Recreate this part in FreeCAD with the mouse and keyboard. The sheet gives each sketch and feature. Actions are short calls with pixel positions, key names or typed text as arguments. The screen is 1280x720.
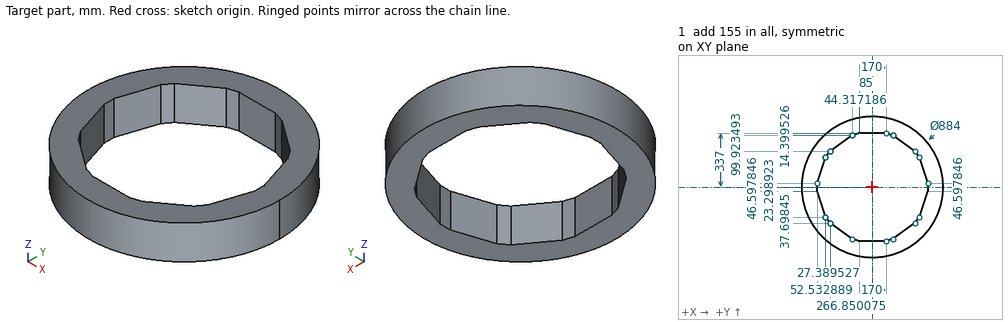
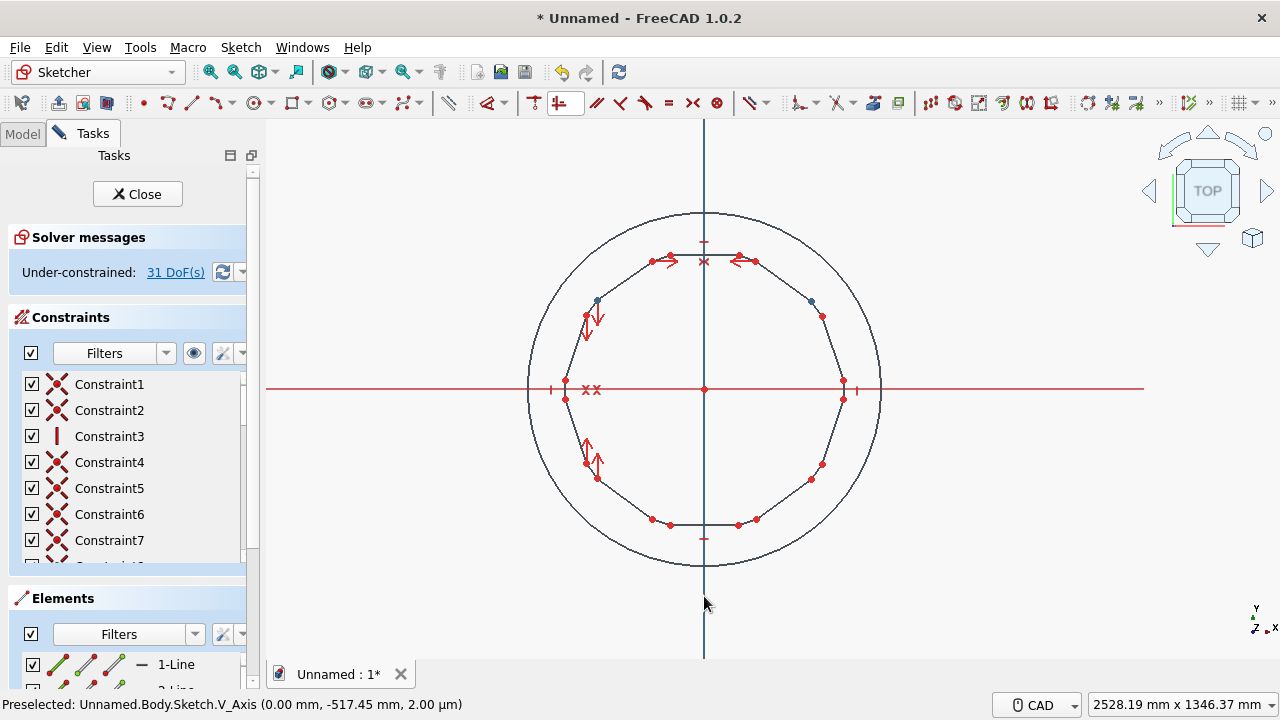
key(s)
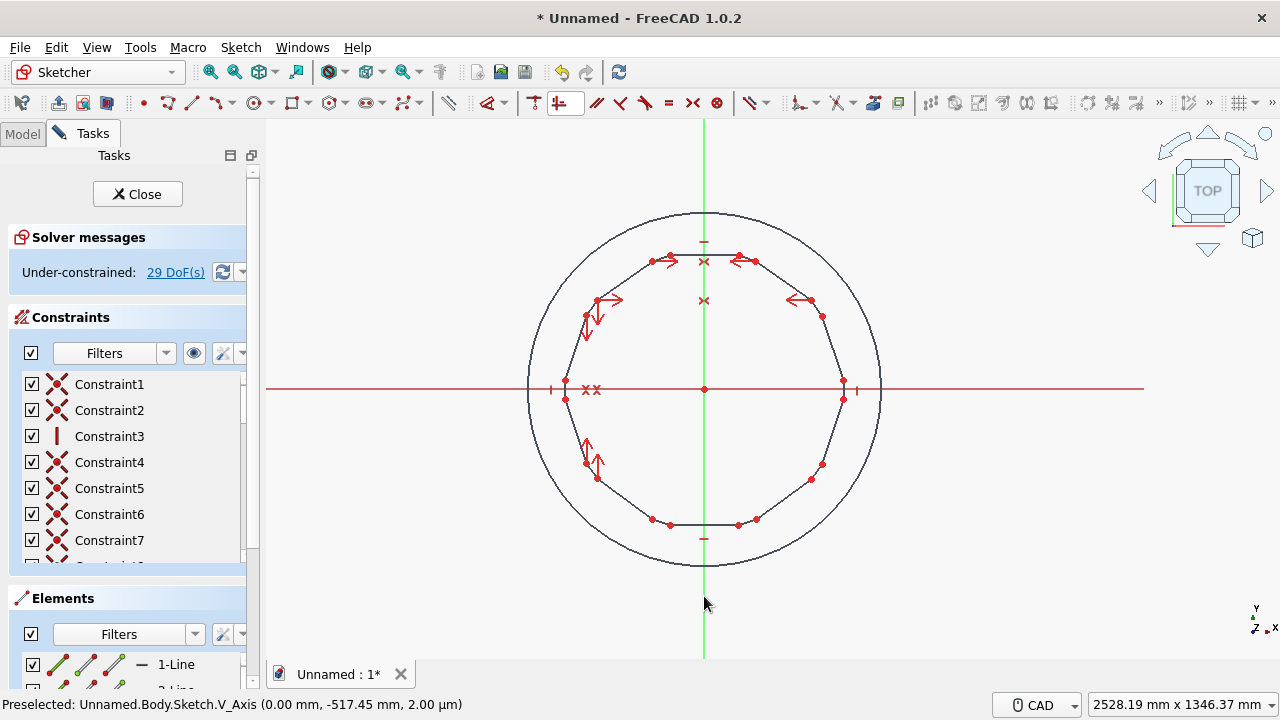
click(587, 315)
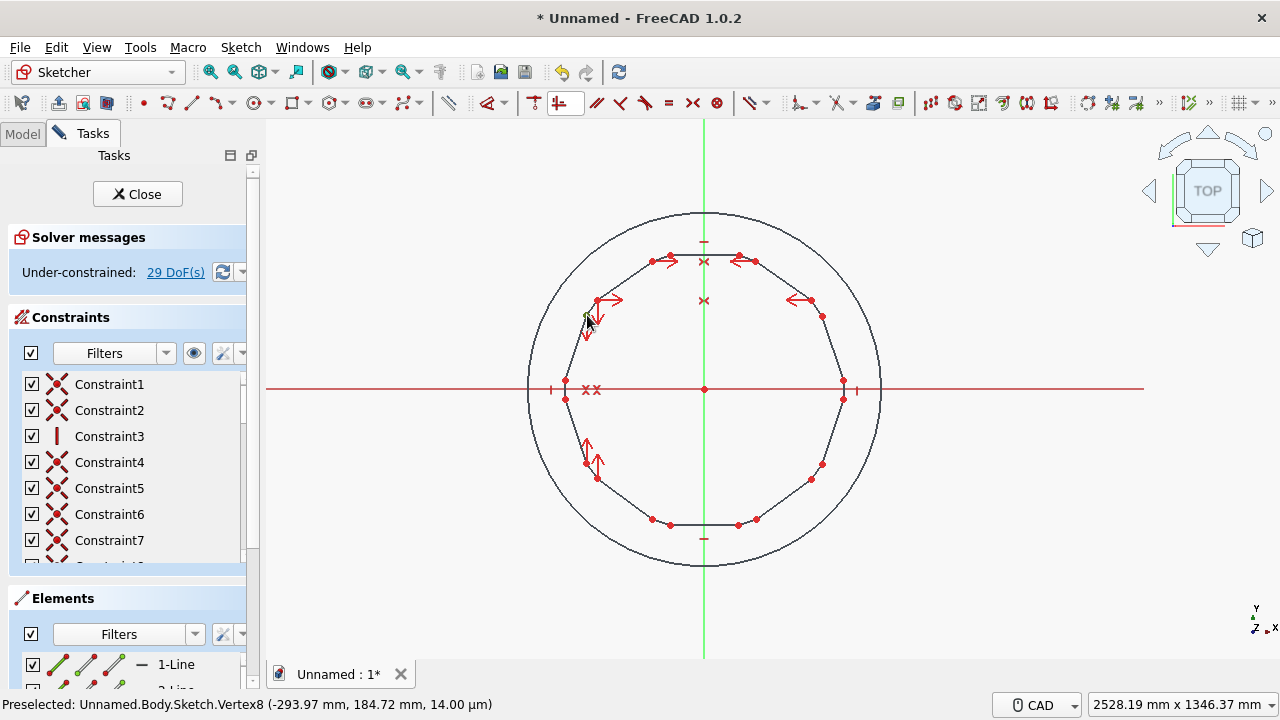
click(822, 316)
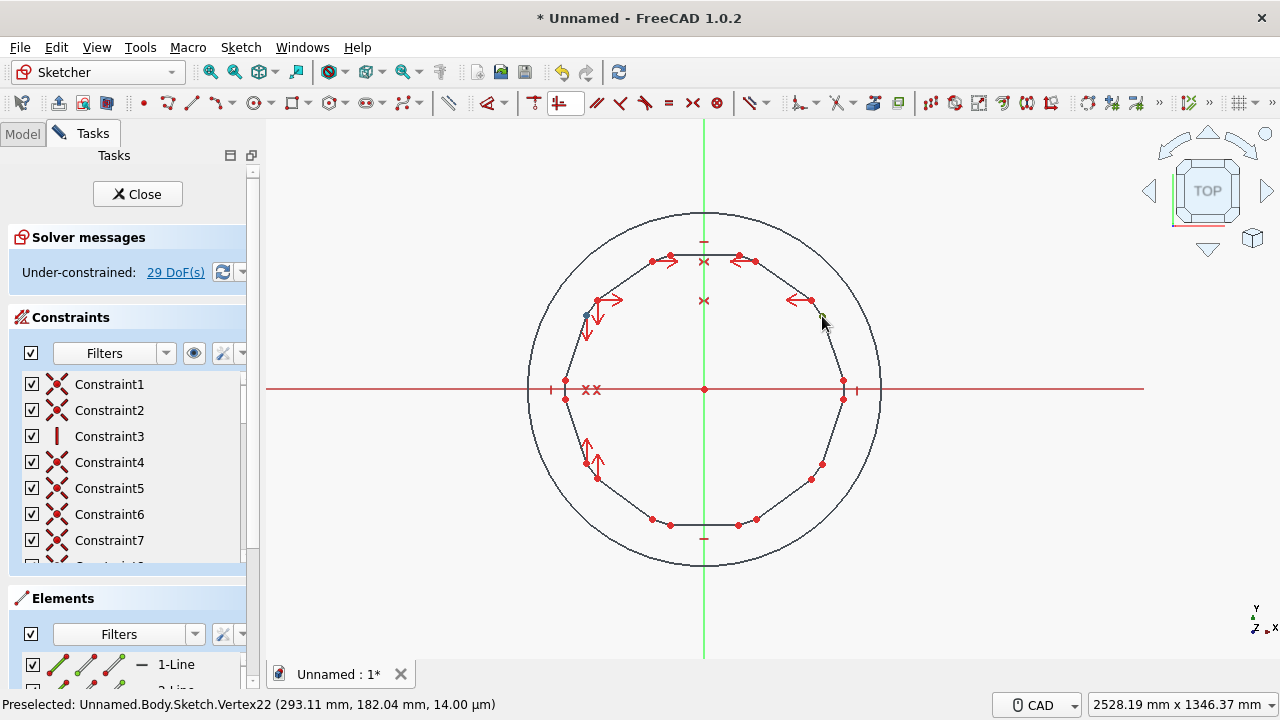
click(704, 596)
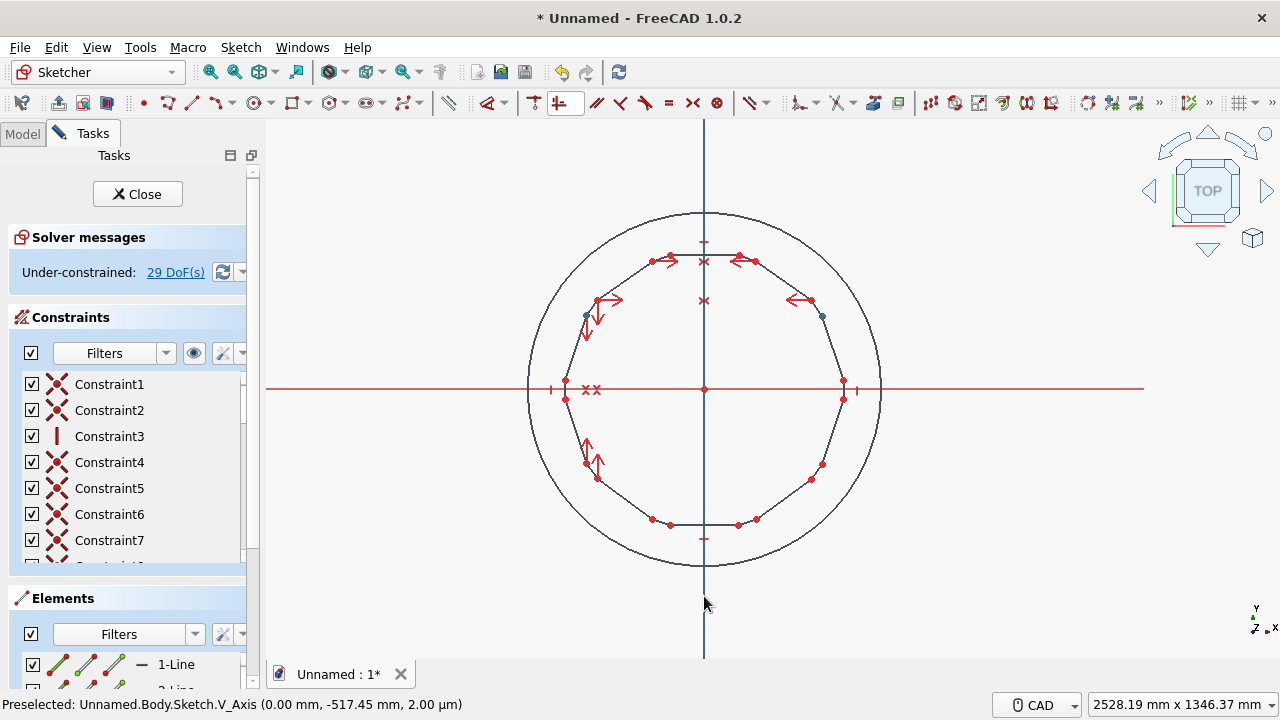
key(s)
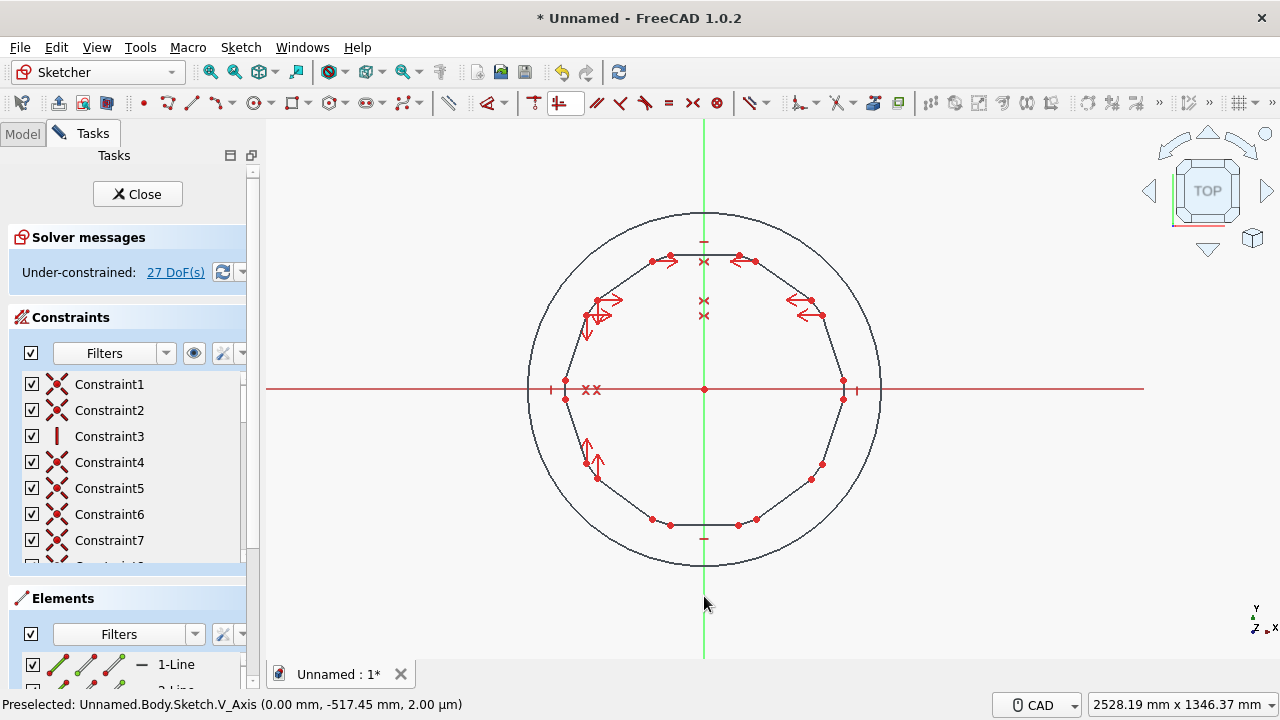
click(565, 381)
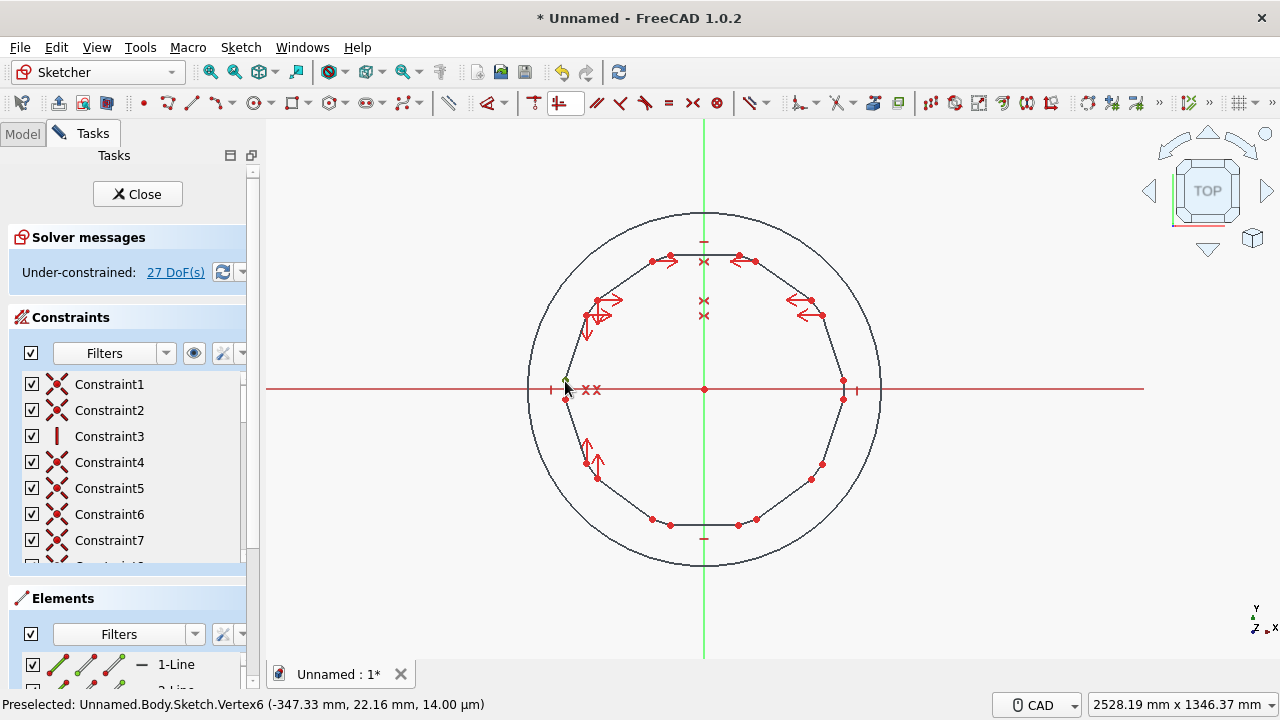
click(844, 381)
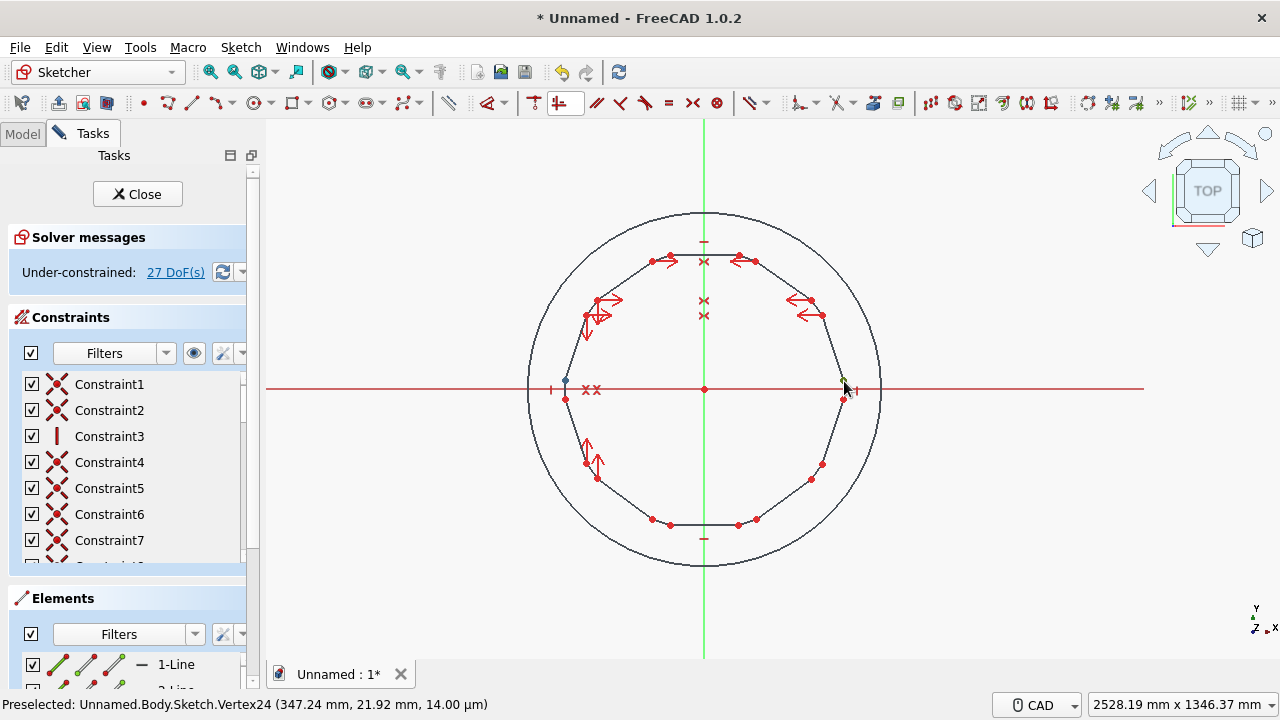
click(704, 596)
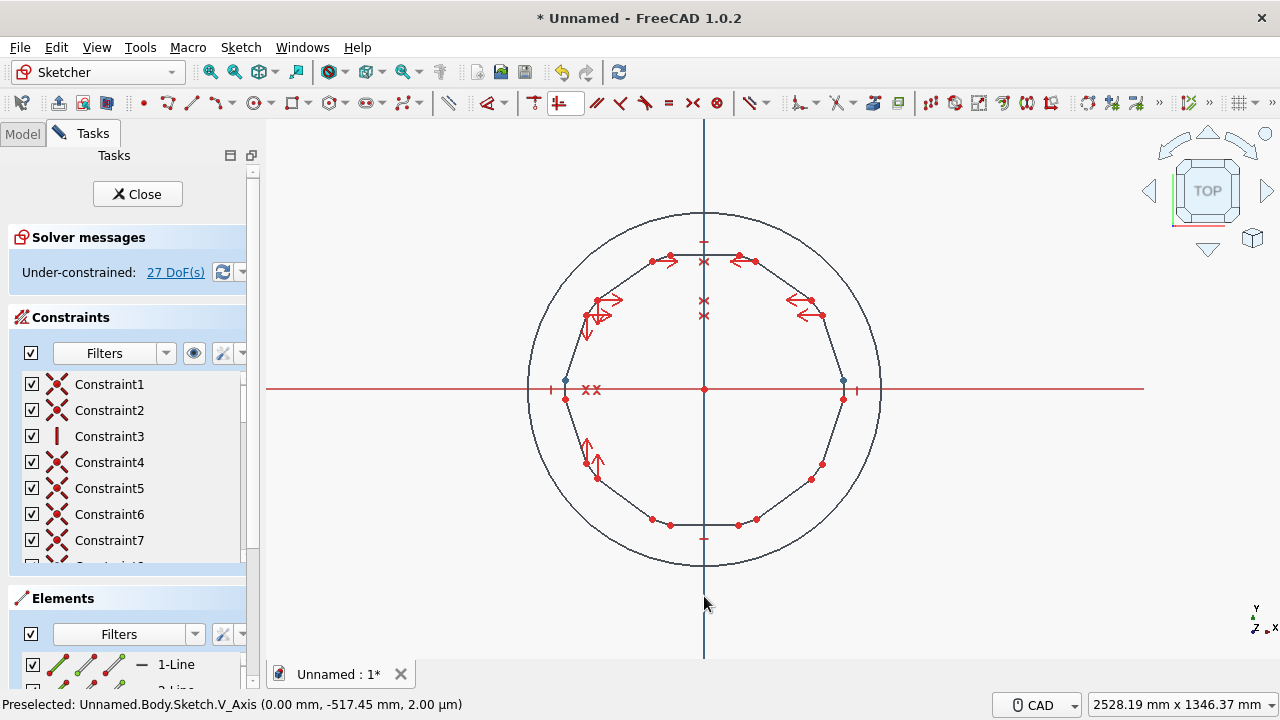
click(694, 104)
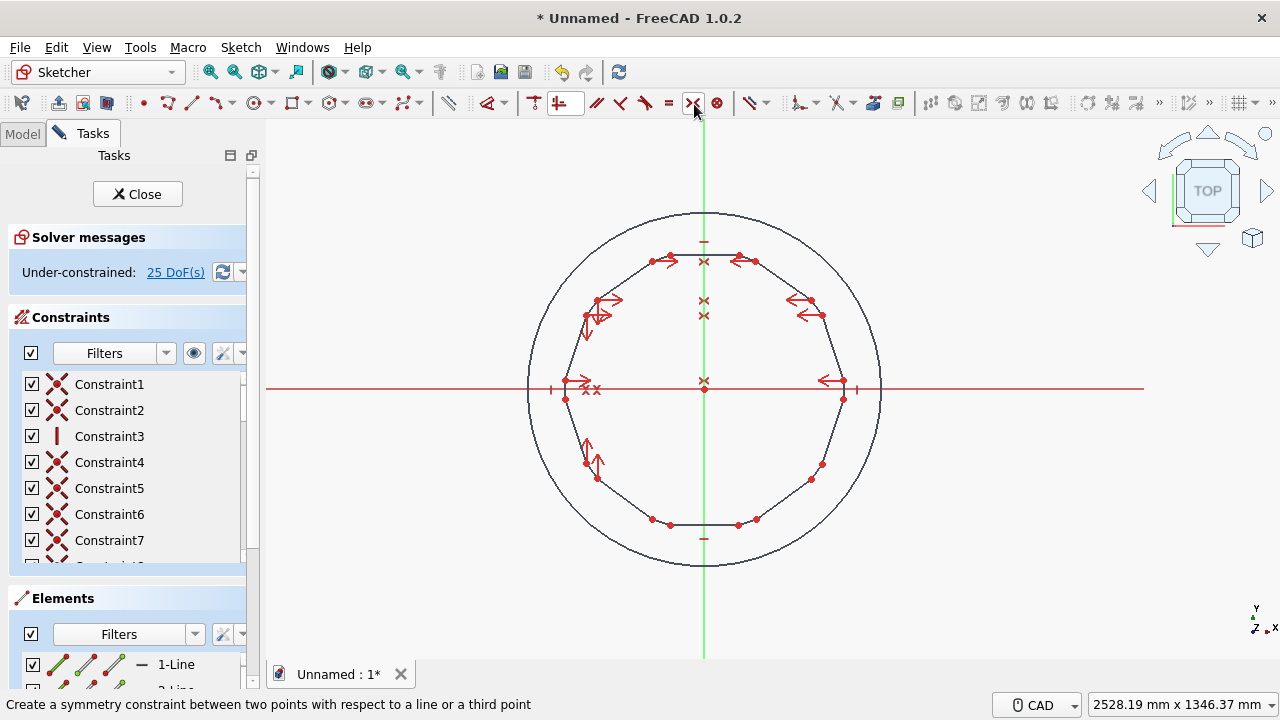
click(587, 464)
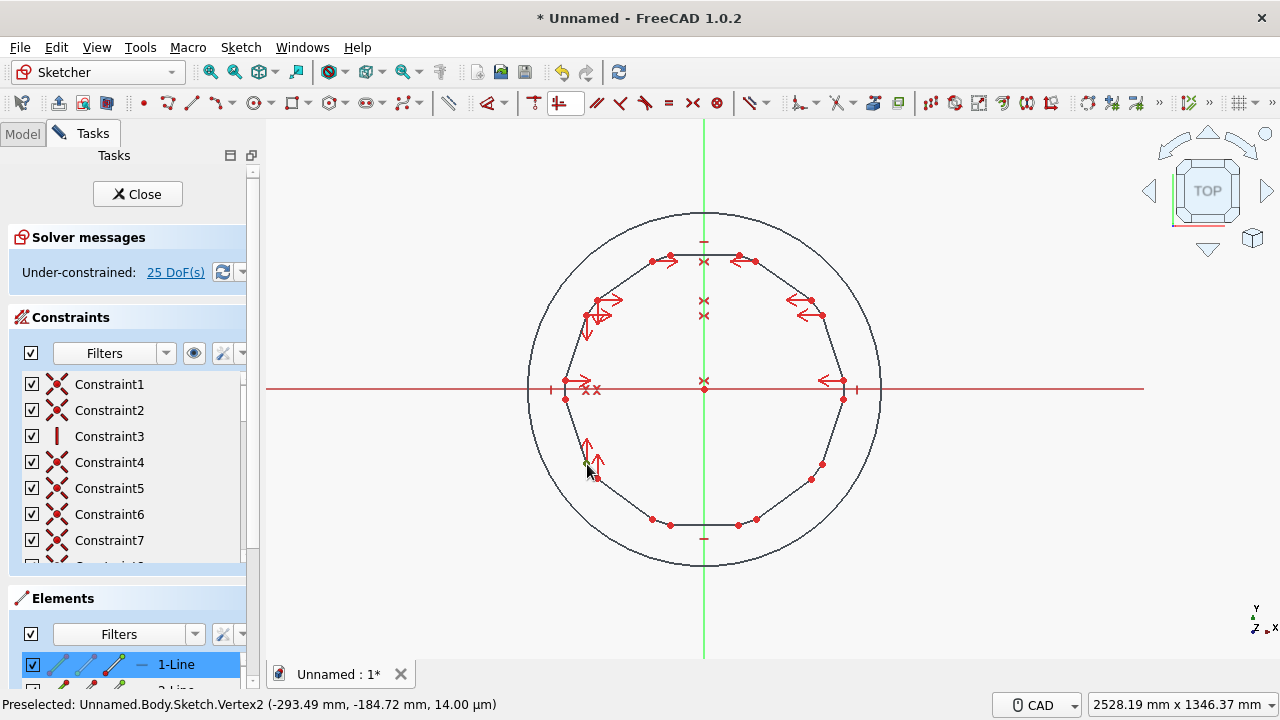
click(822, 464)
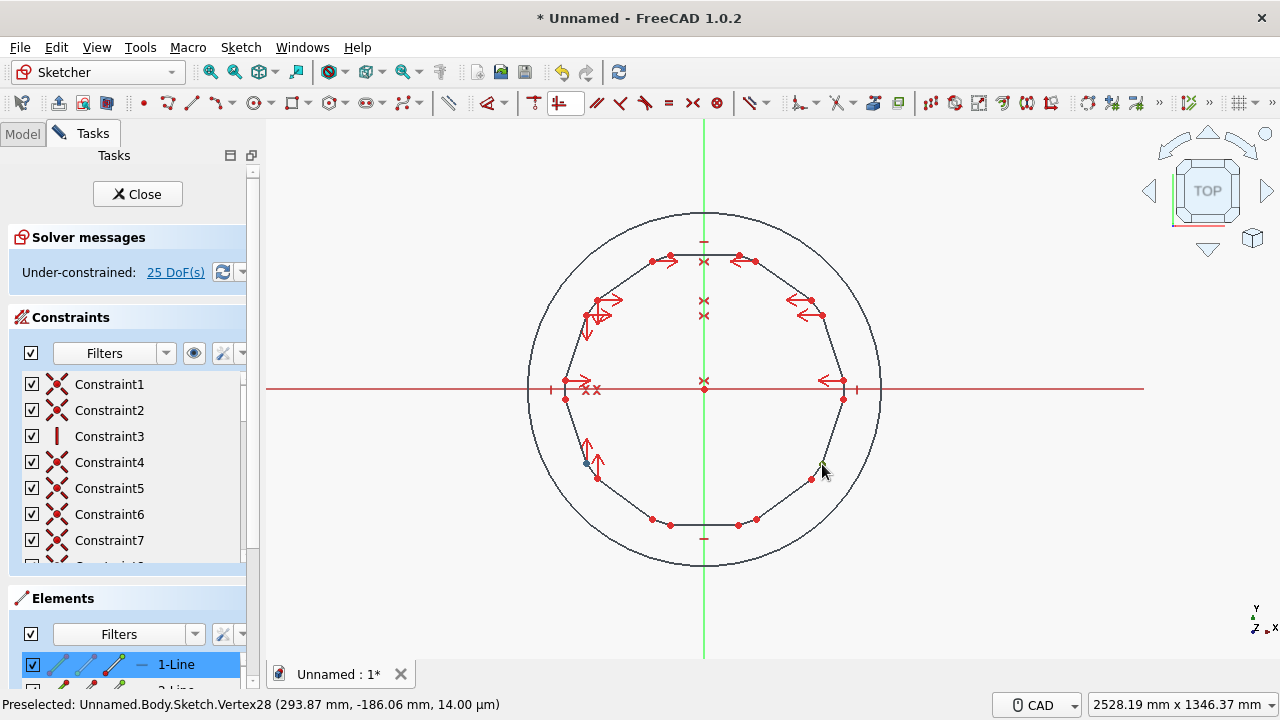
click(704, 596)